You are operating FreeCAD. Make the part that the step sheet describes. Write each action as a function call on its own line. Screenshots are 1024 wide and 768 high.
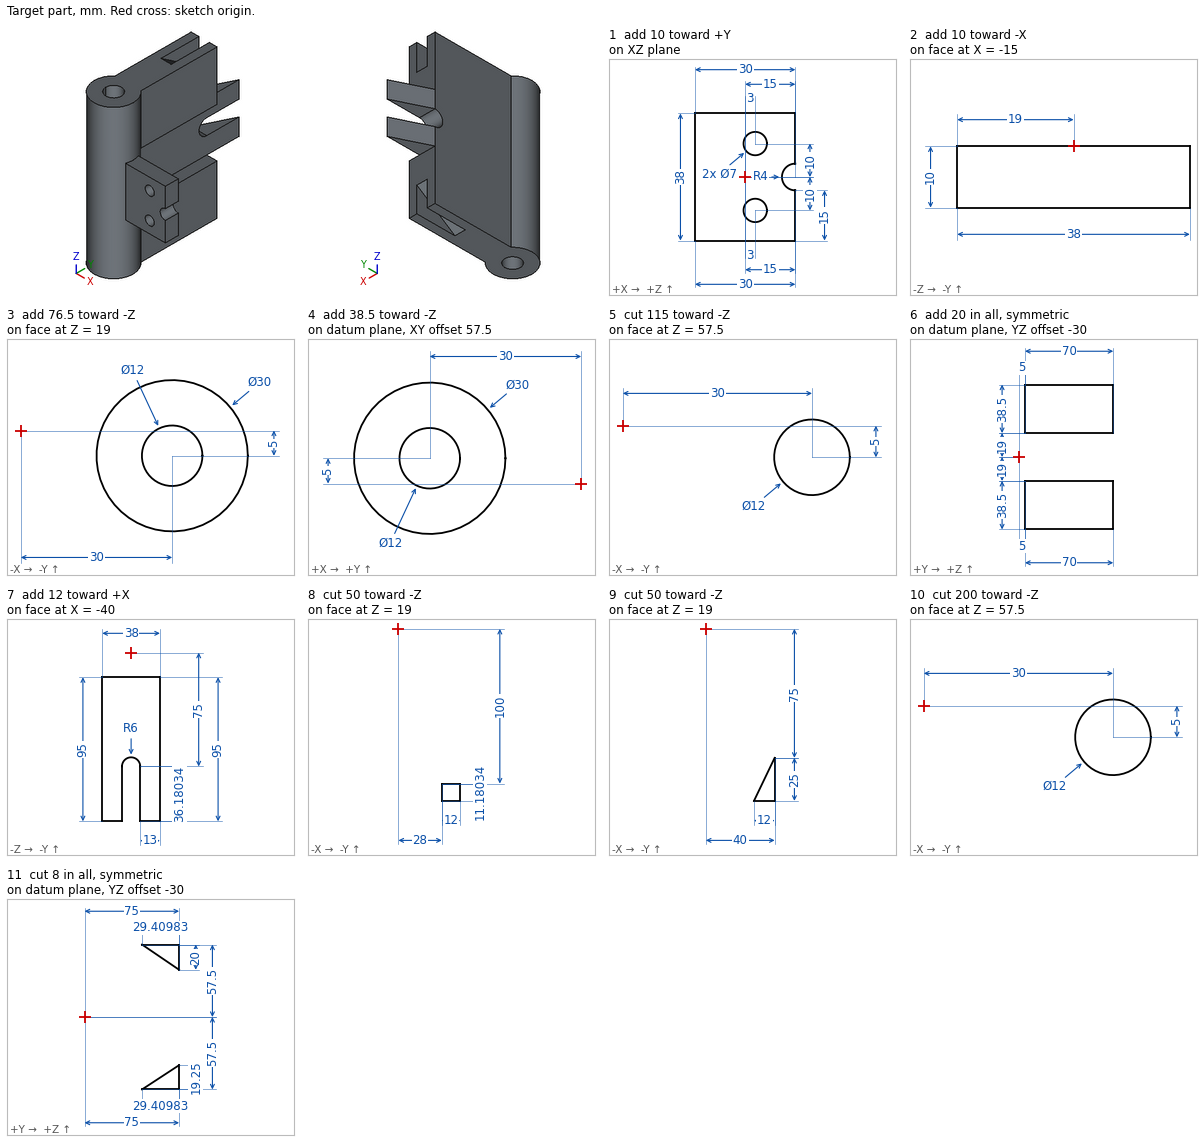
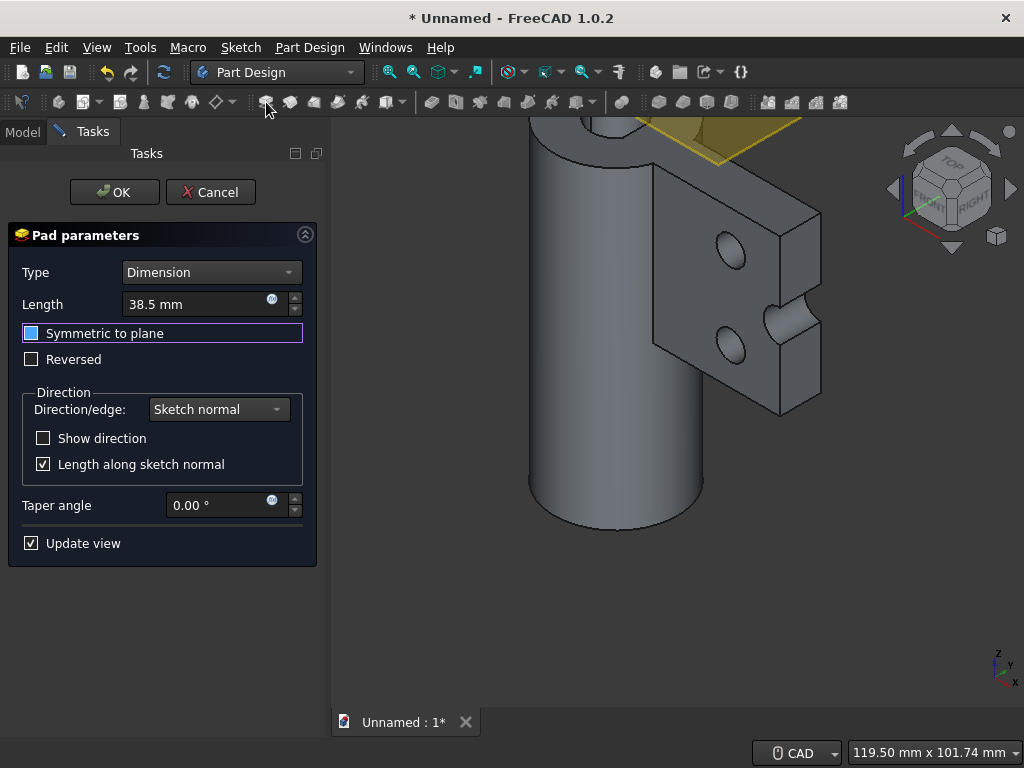
click(30, 359)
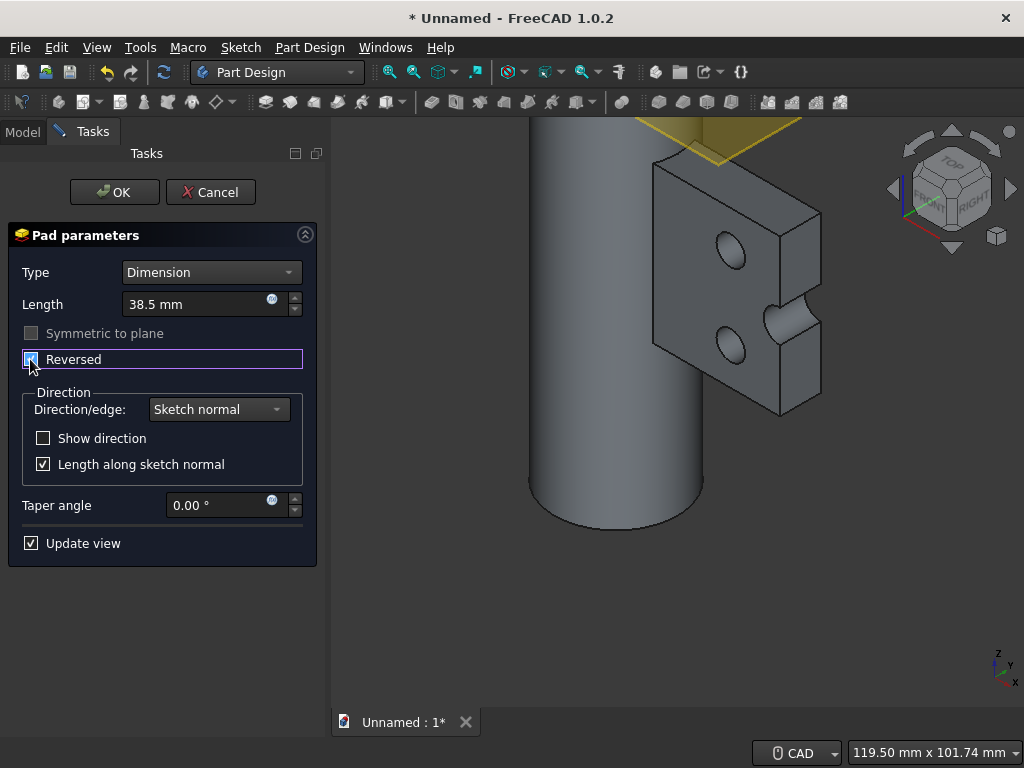
click(115, 192)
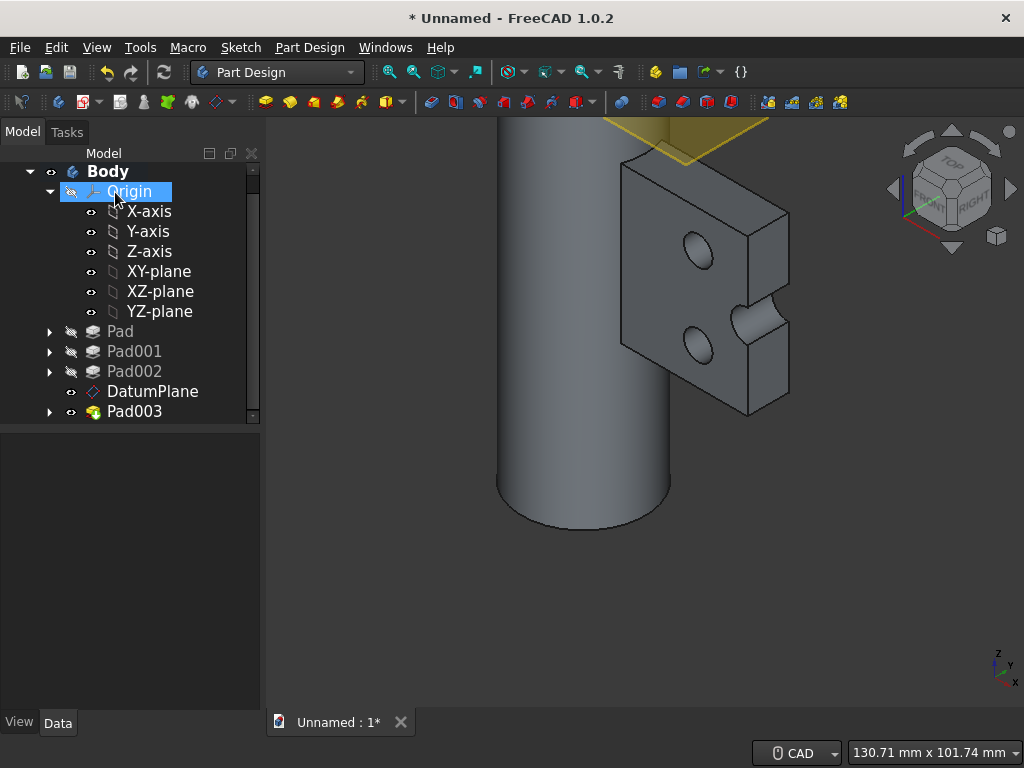
click(116, 392)
key(space)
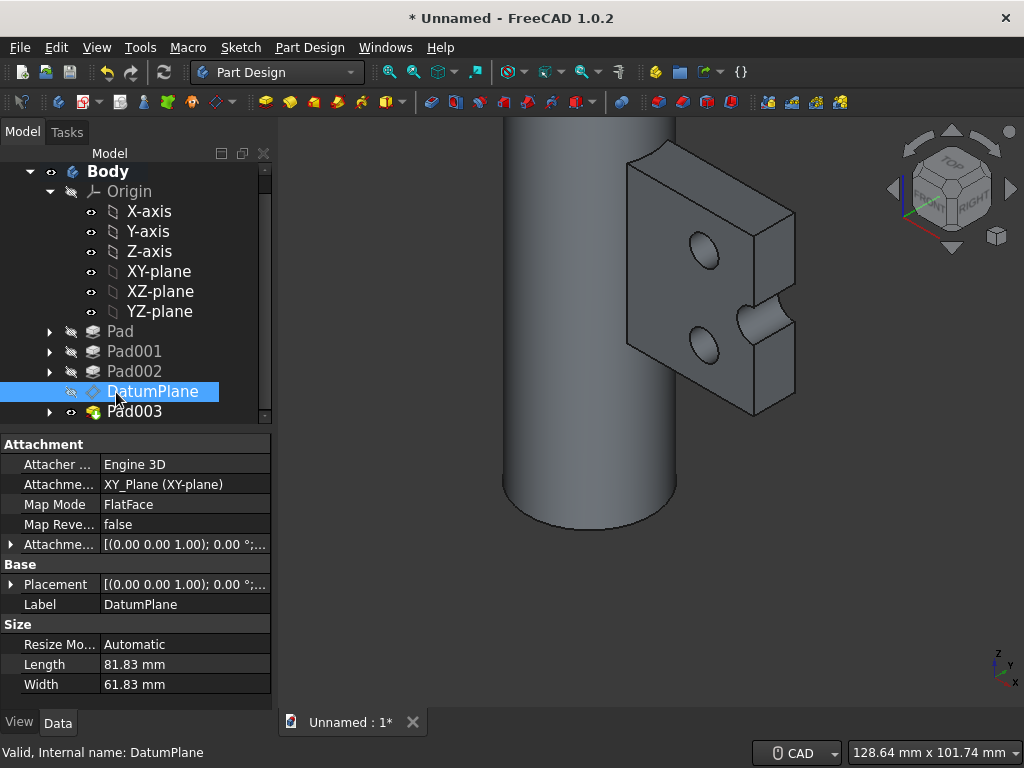
click(390, 72)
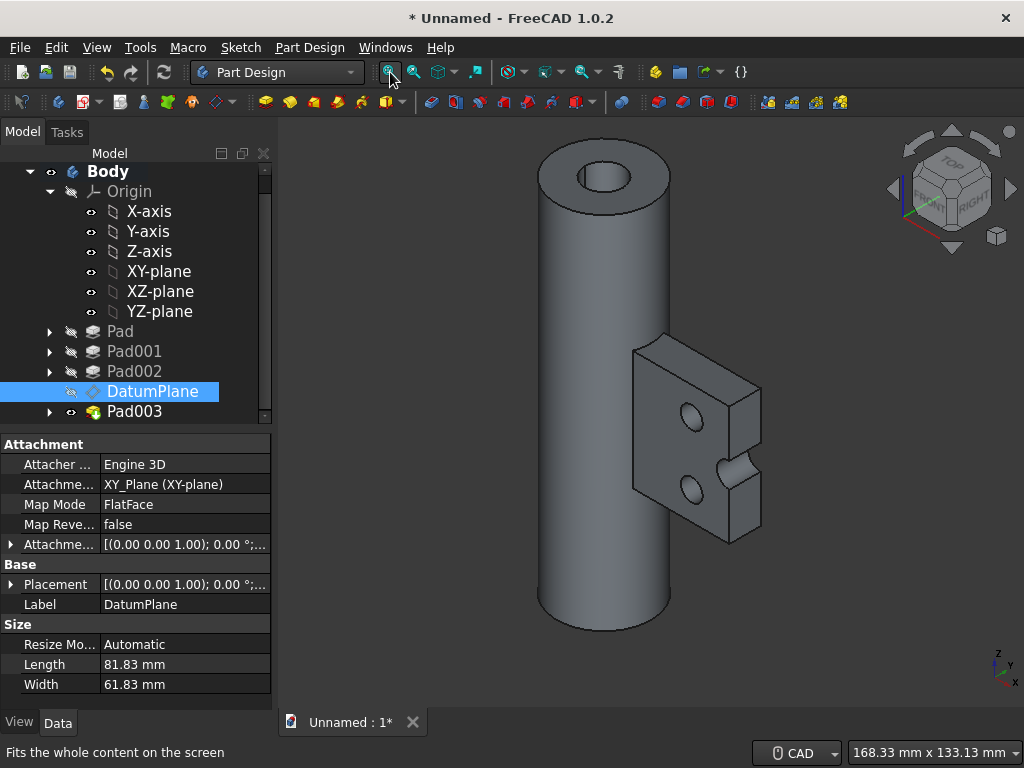
click(644, 184)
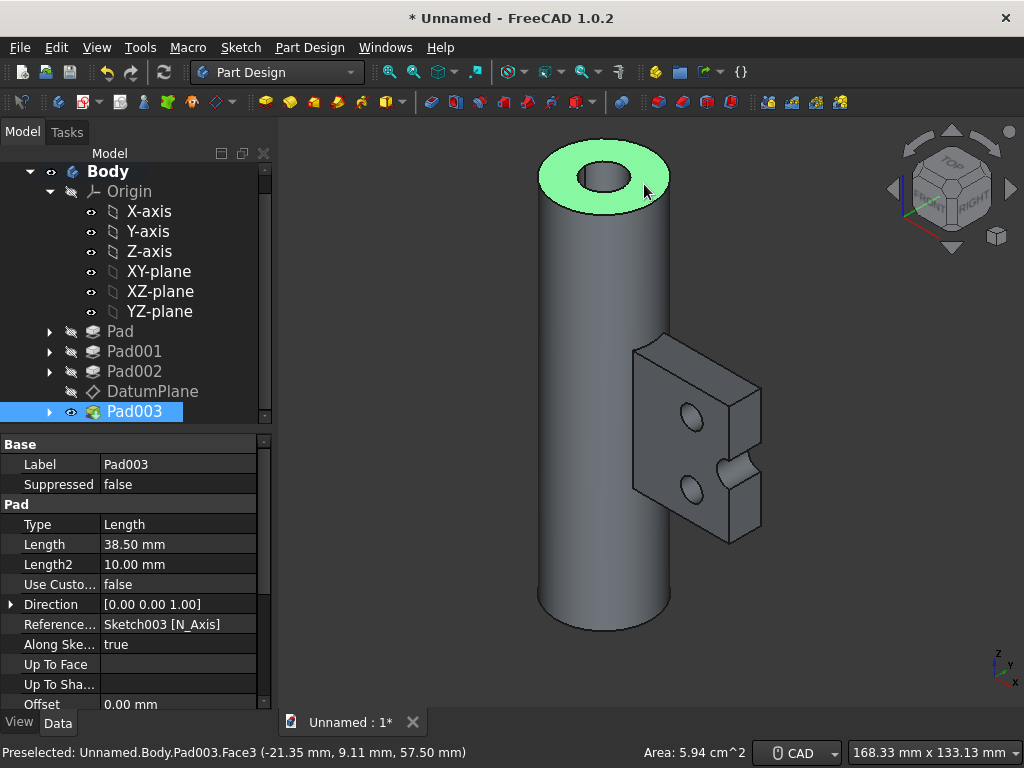
click(84, 102)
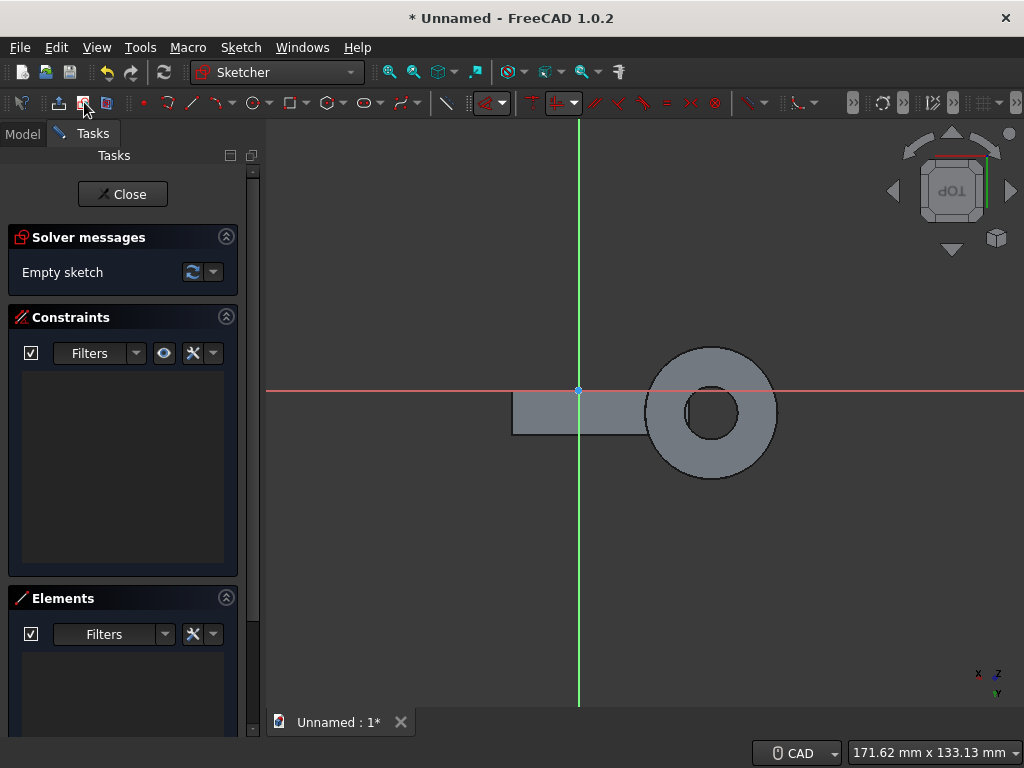
scroll(732, 413, up, 10)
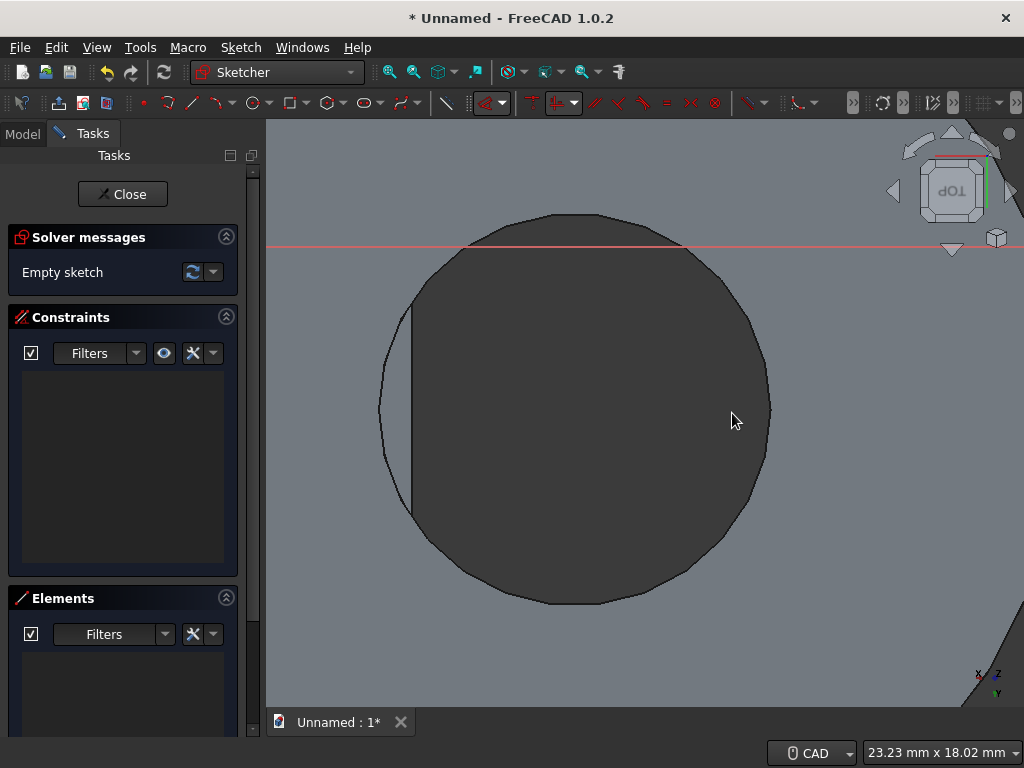
click(254, 104)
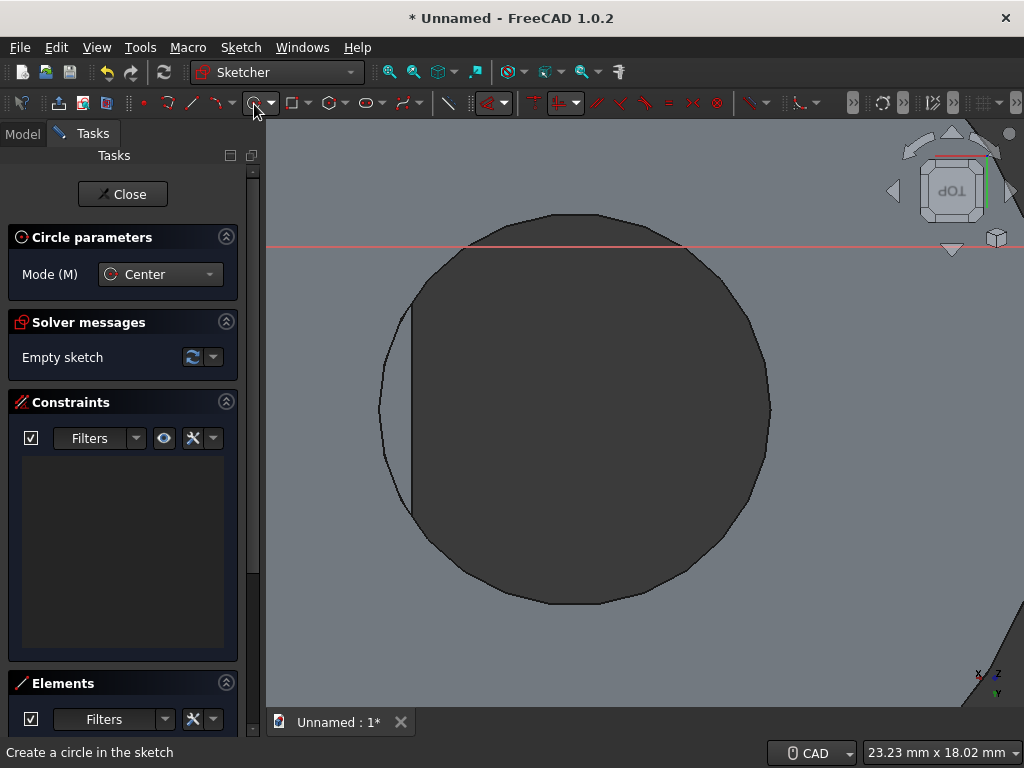
click(575, 410)
click(713, 271)
key(Escape)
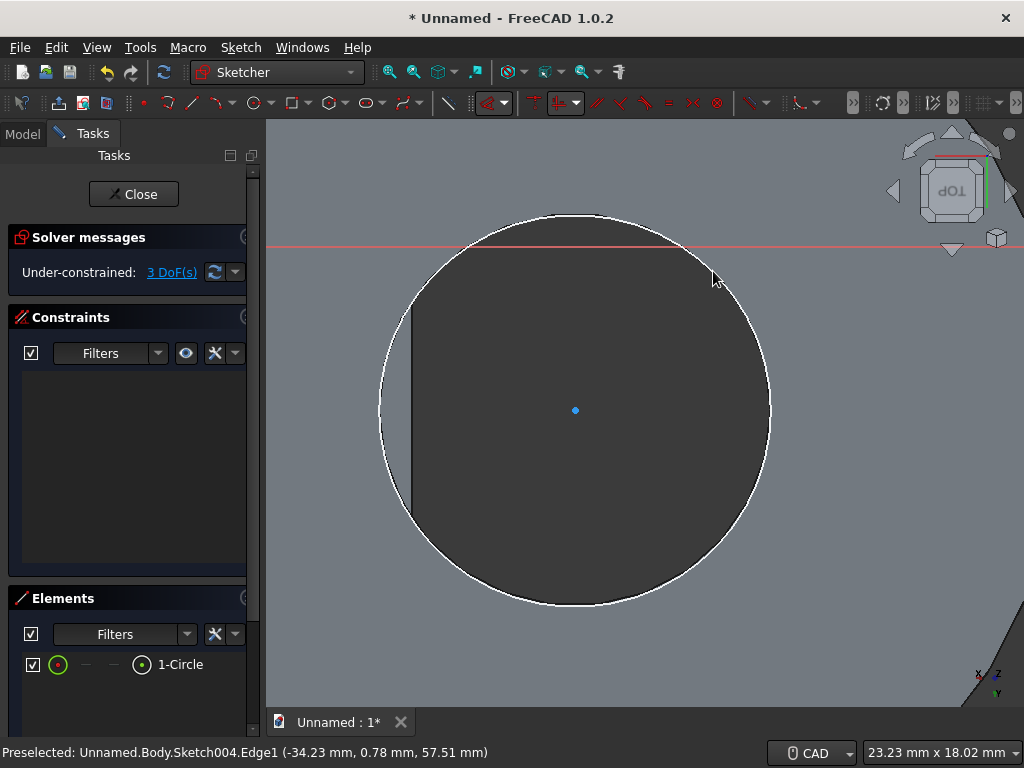
click(713, 272)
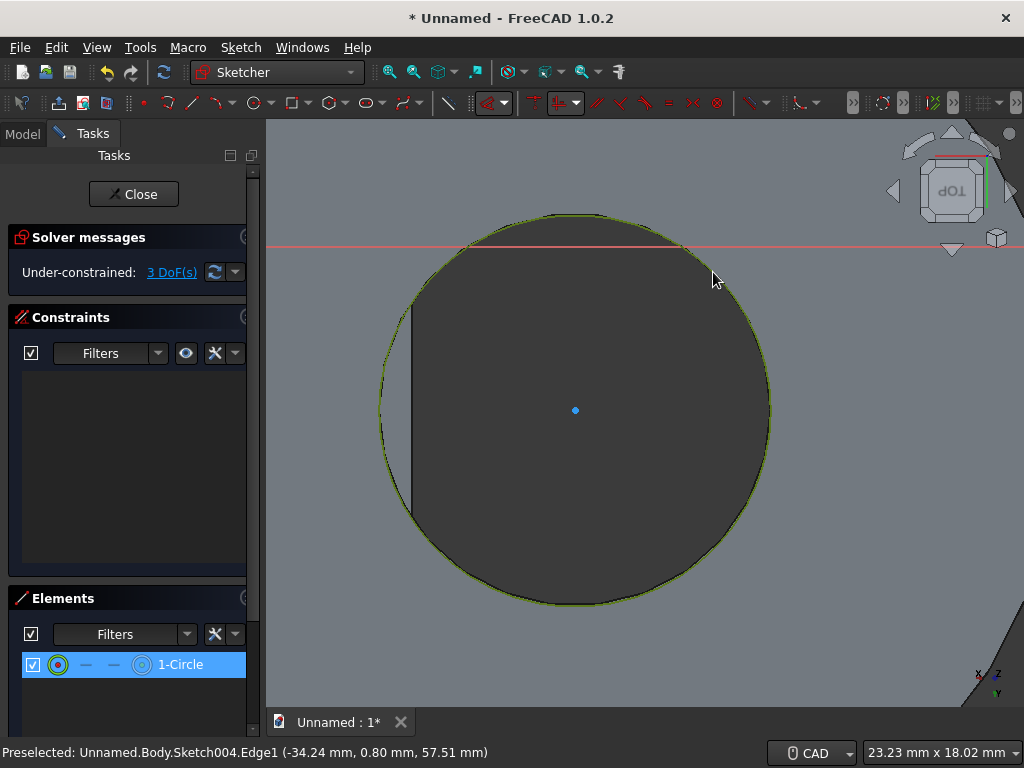
click(506, 104)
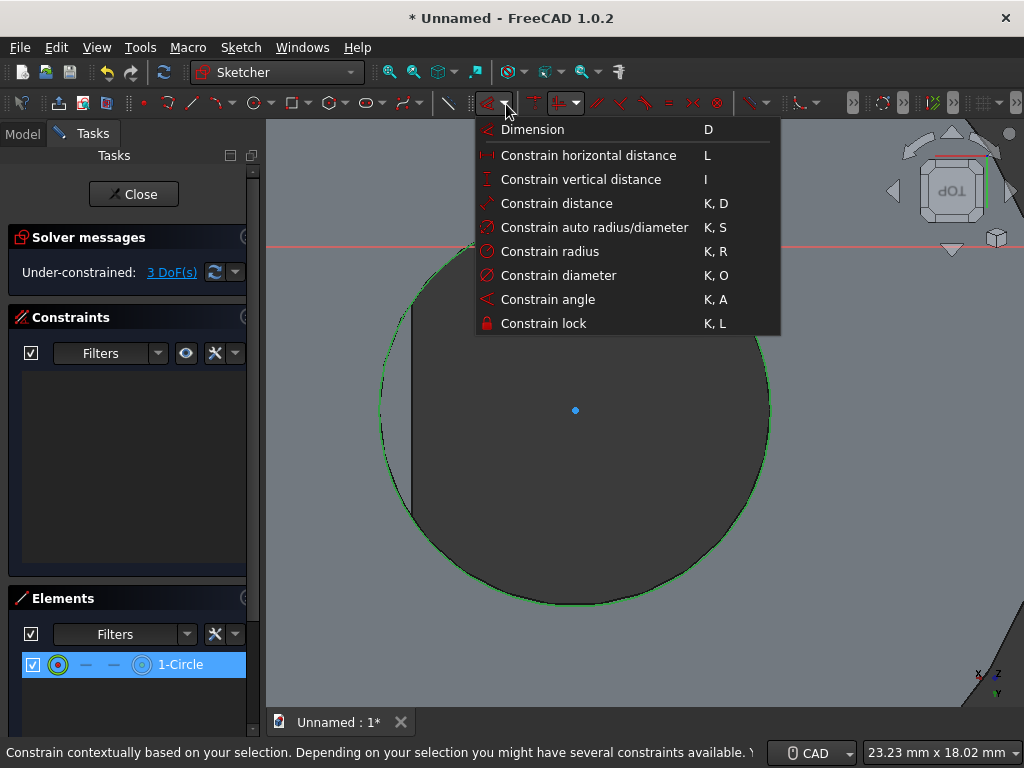
click(628, 275)